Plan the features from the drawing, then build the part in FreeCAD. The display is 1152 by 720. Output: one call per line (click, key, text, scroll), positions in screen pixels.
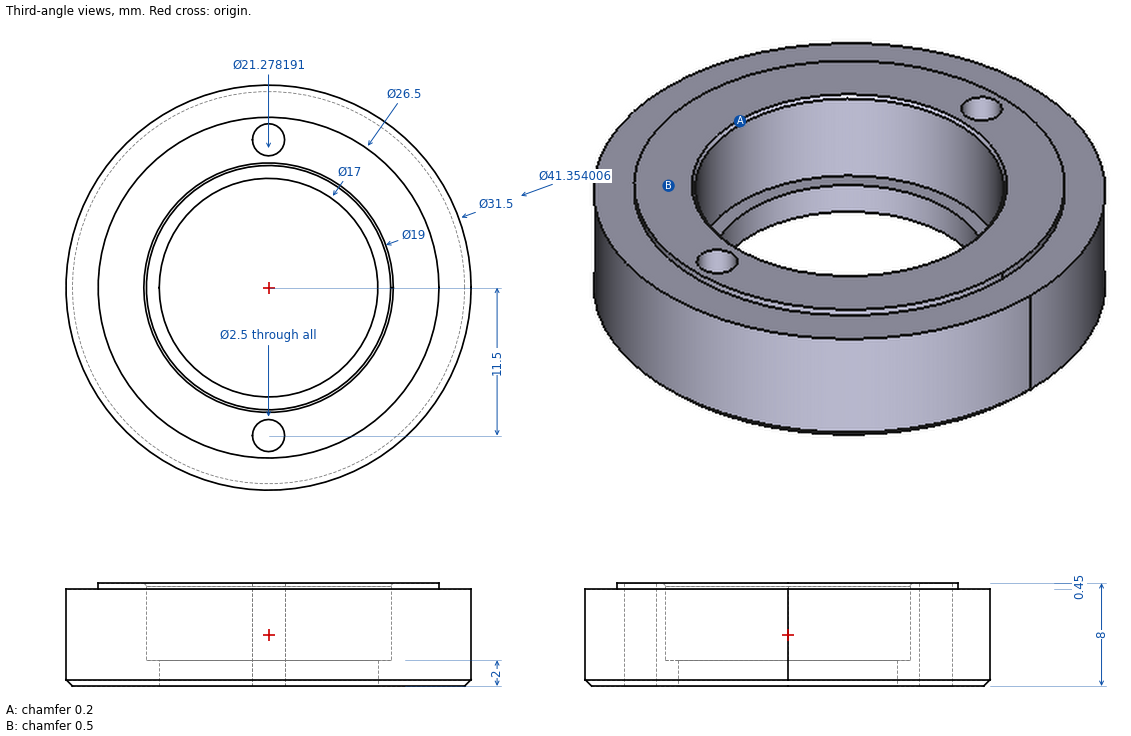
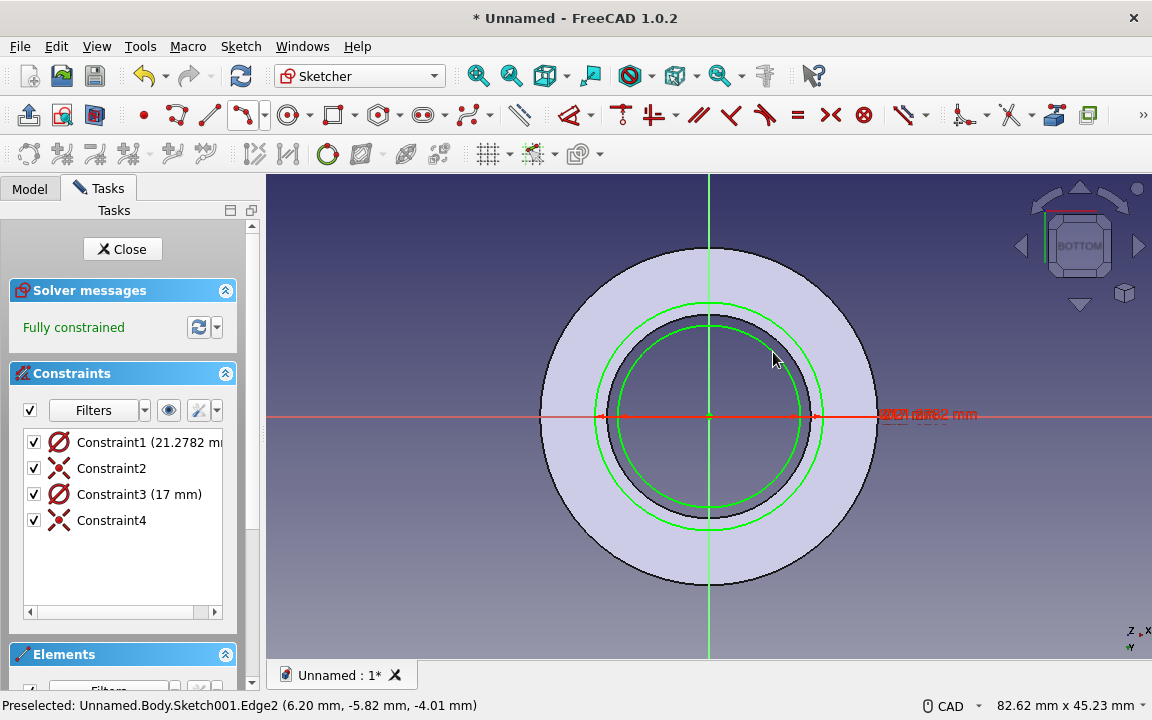
click(123, 249)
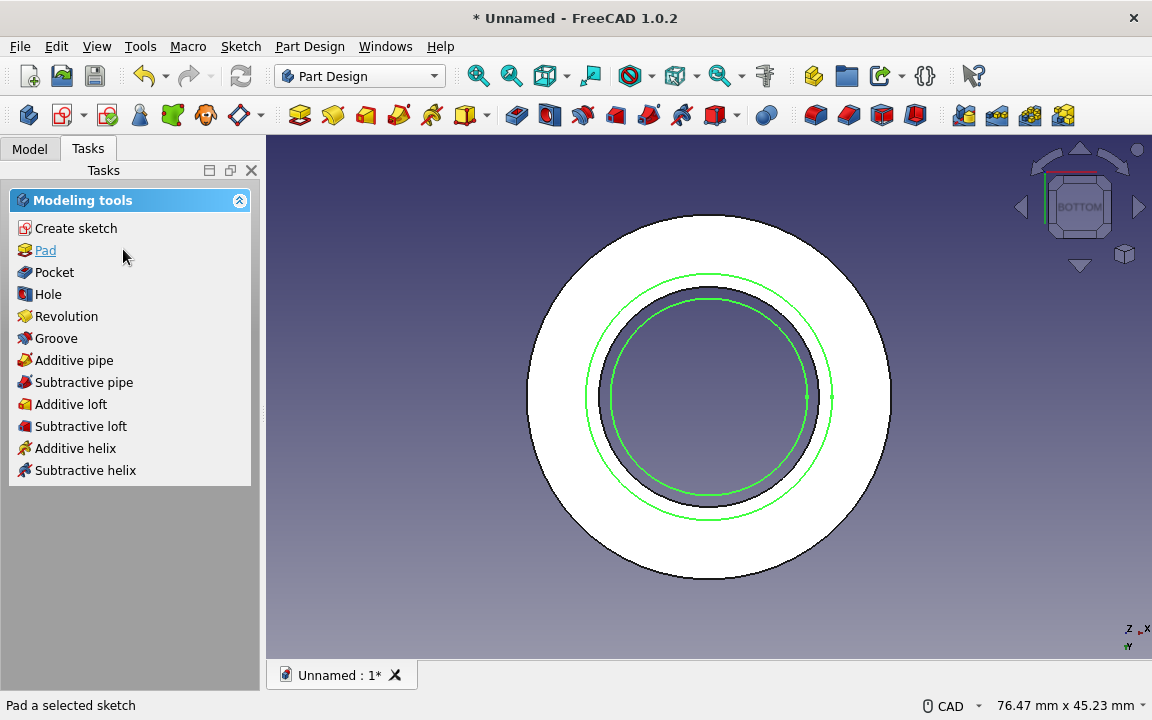
click(300, 116)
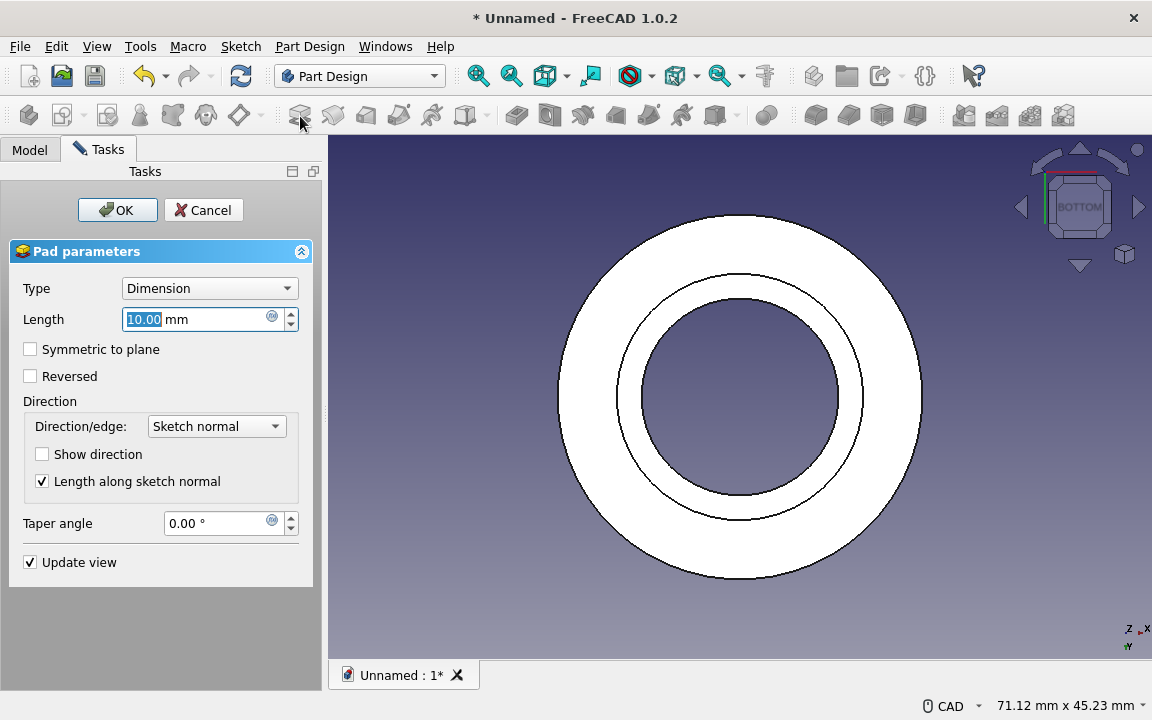
text(2)
key(Tab)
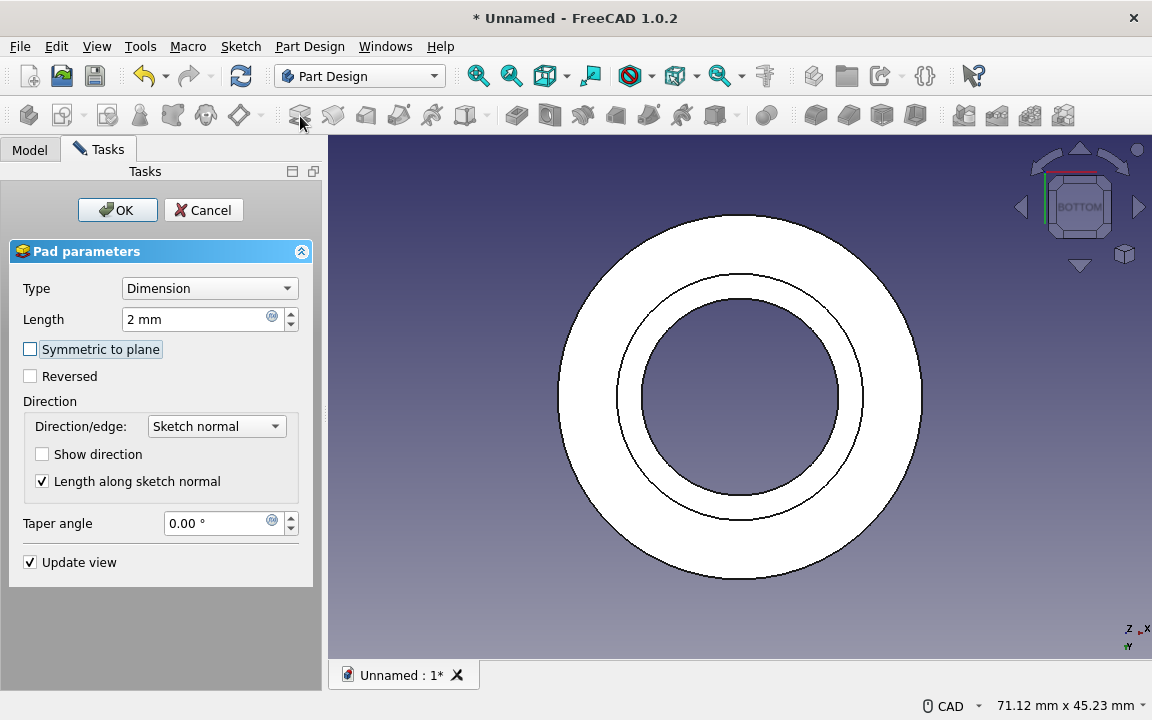
click(31, 376)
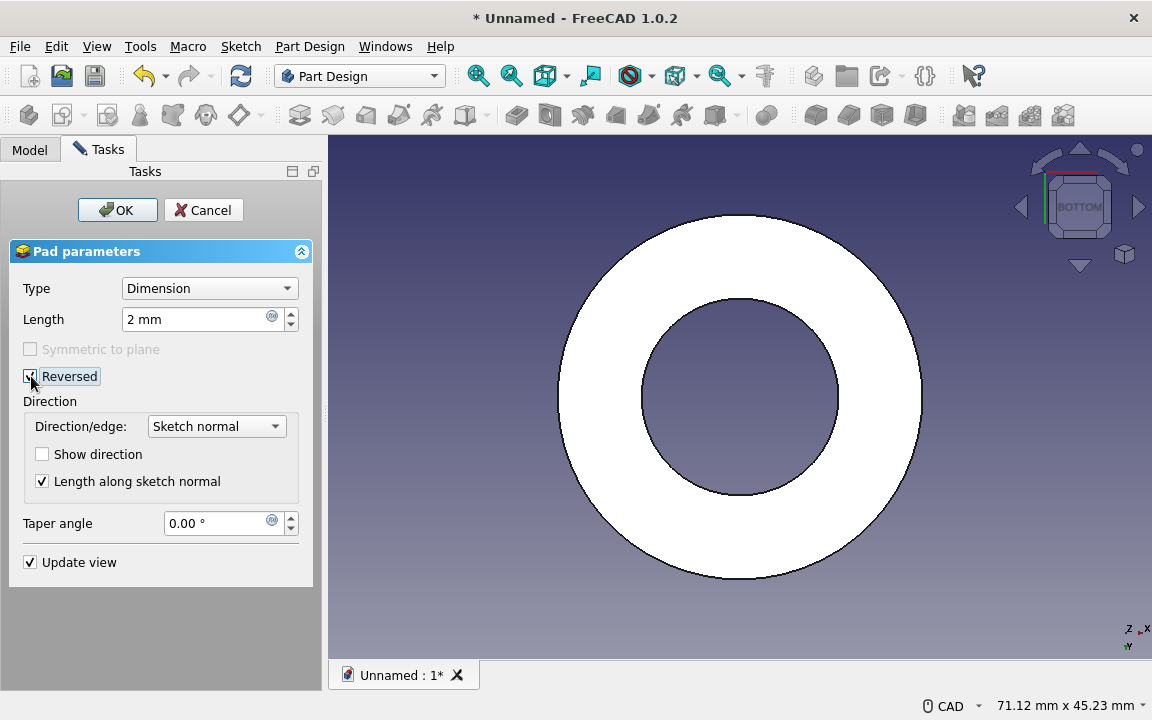
click(118, 210)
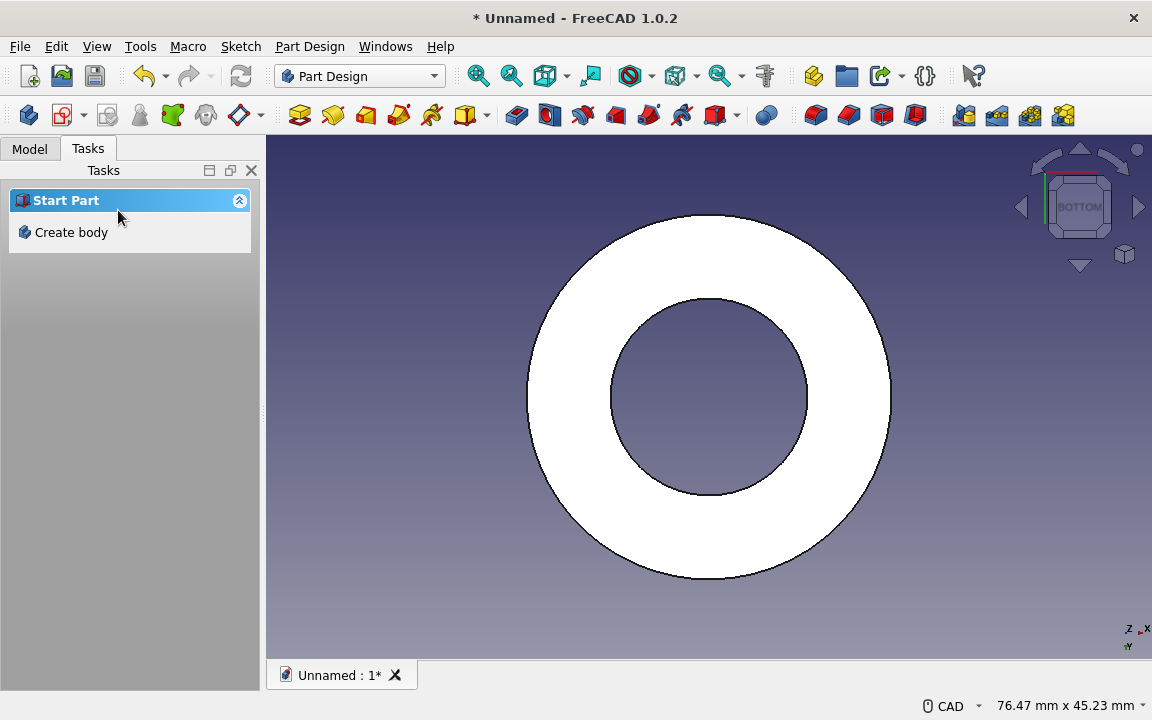
key(0)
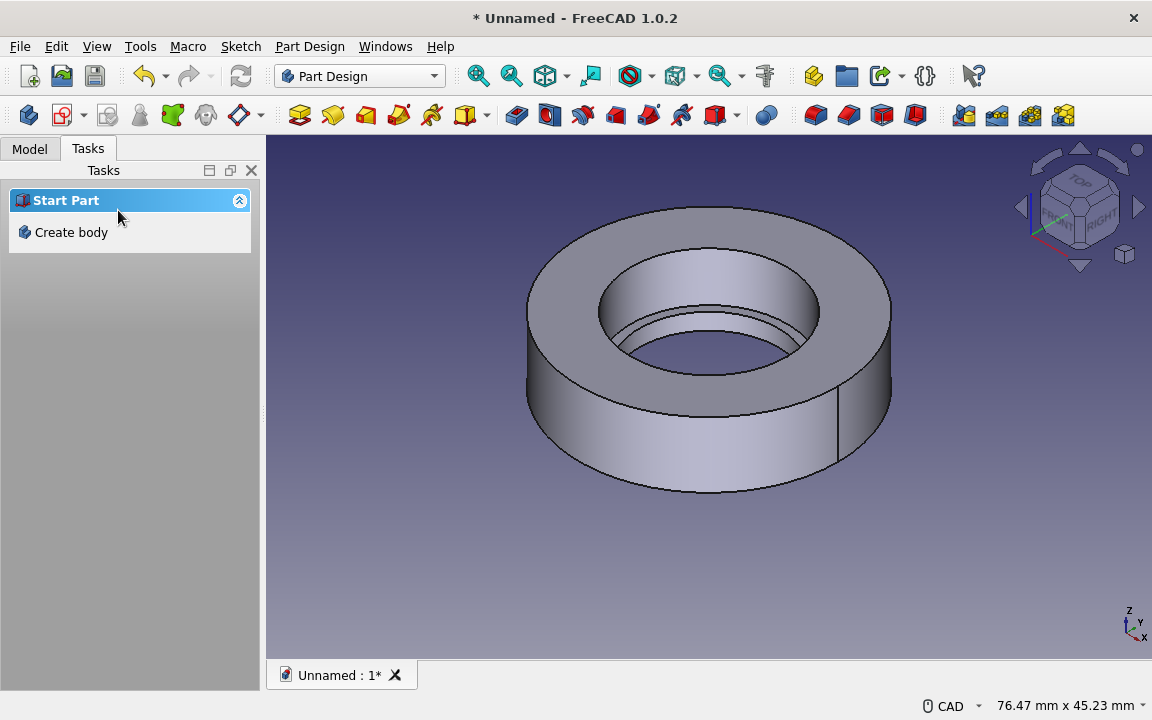
click(562, 311)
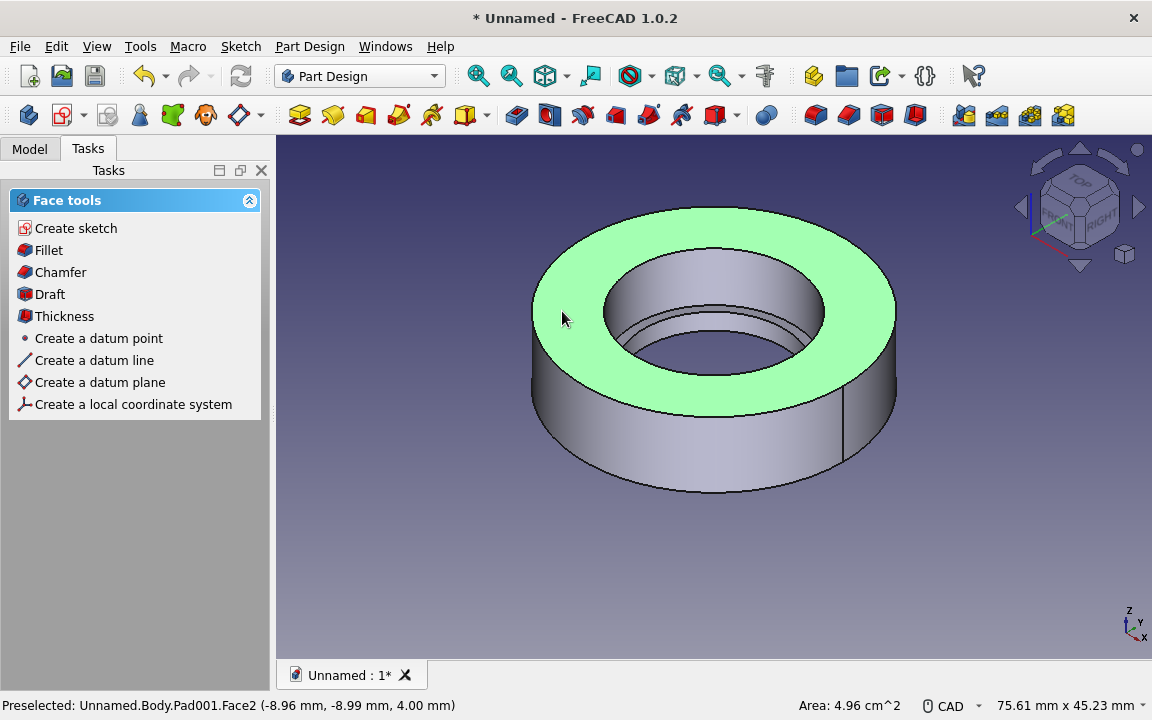
click(62, 116)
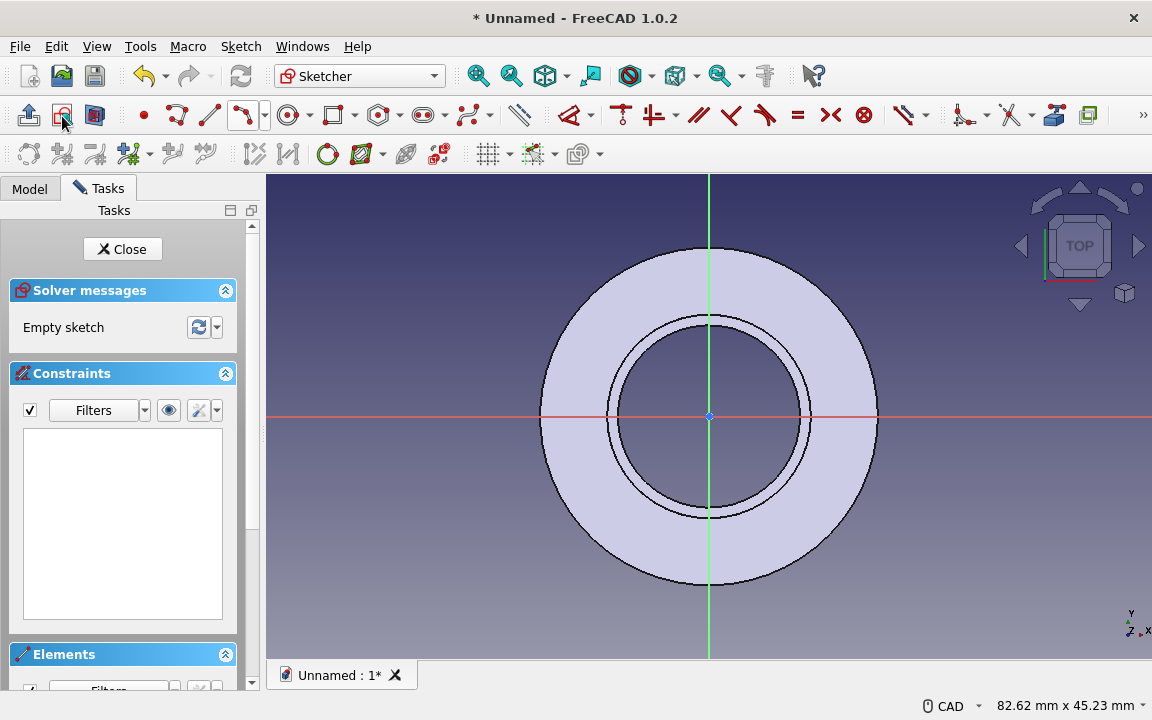
scroll(716, 552, up, 12)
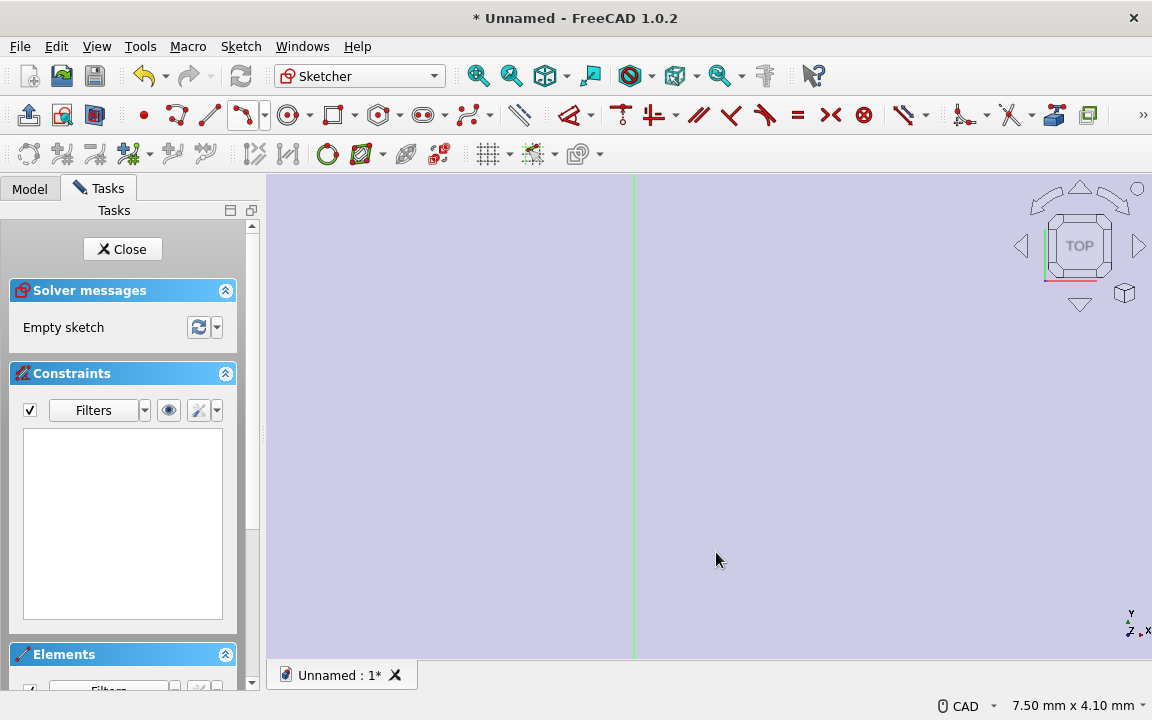
click(288, 116)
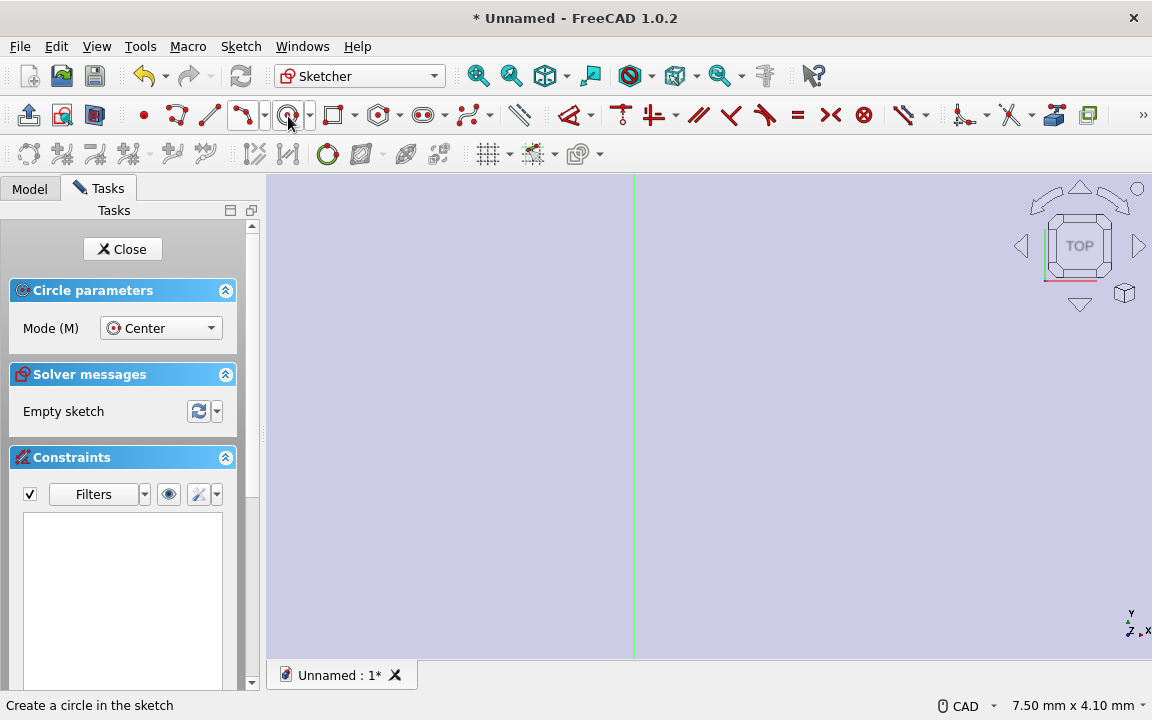
click(634, 410)
move(738, 305)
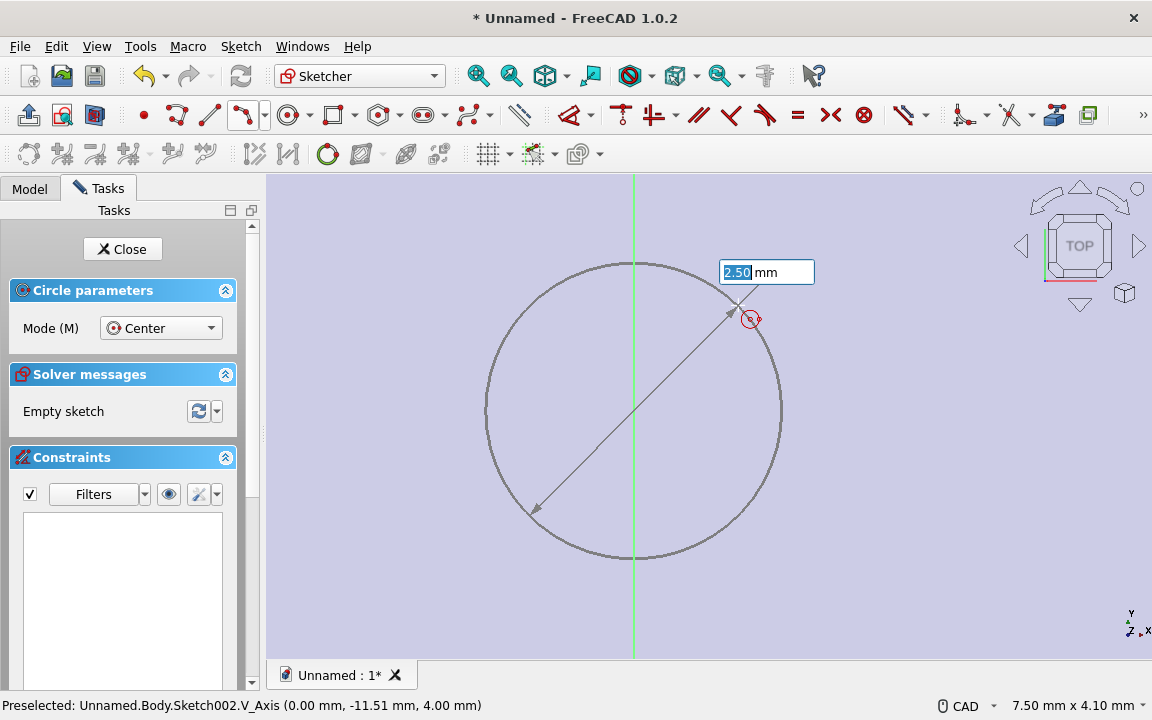
text(2.5)
key(Return)
key(Escape)